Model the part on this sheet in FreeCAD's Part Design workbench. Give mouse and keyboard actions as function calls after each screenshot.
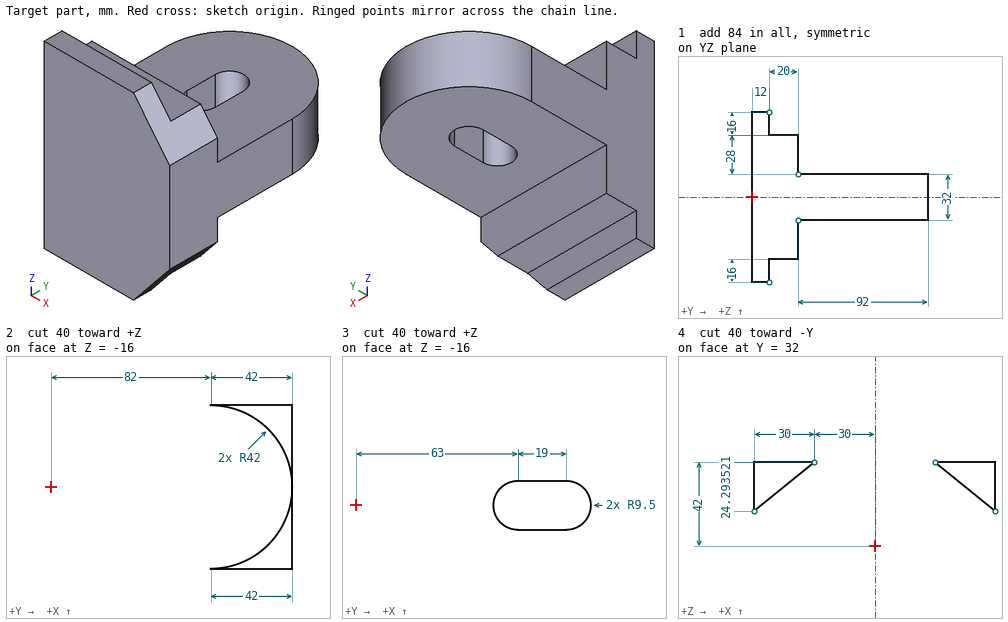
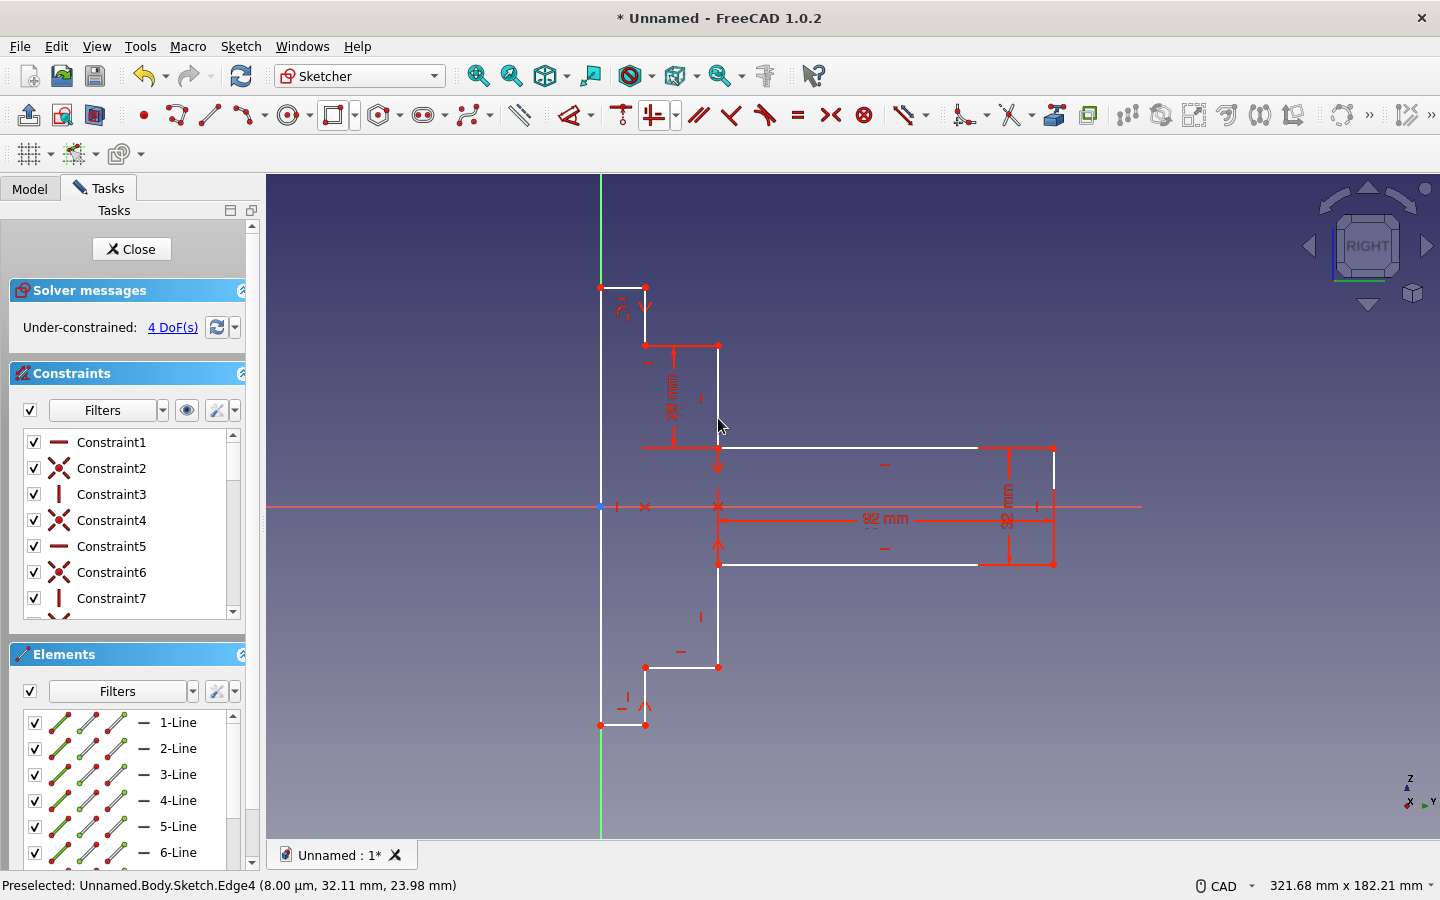
click(696, 346)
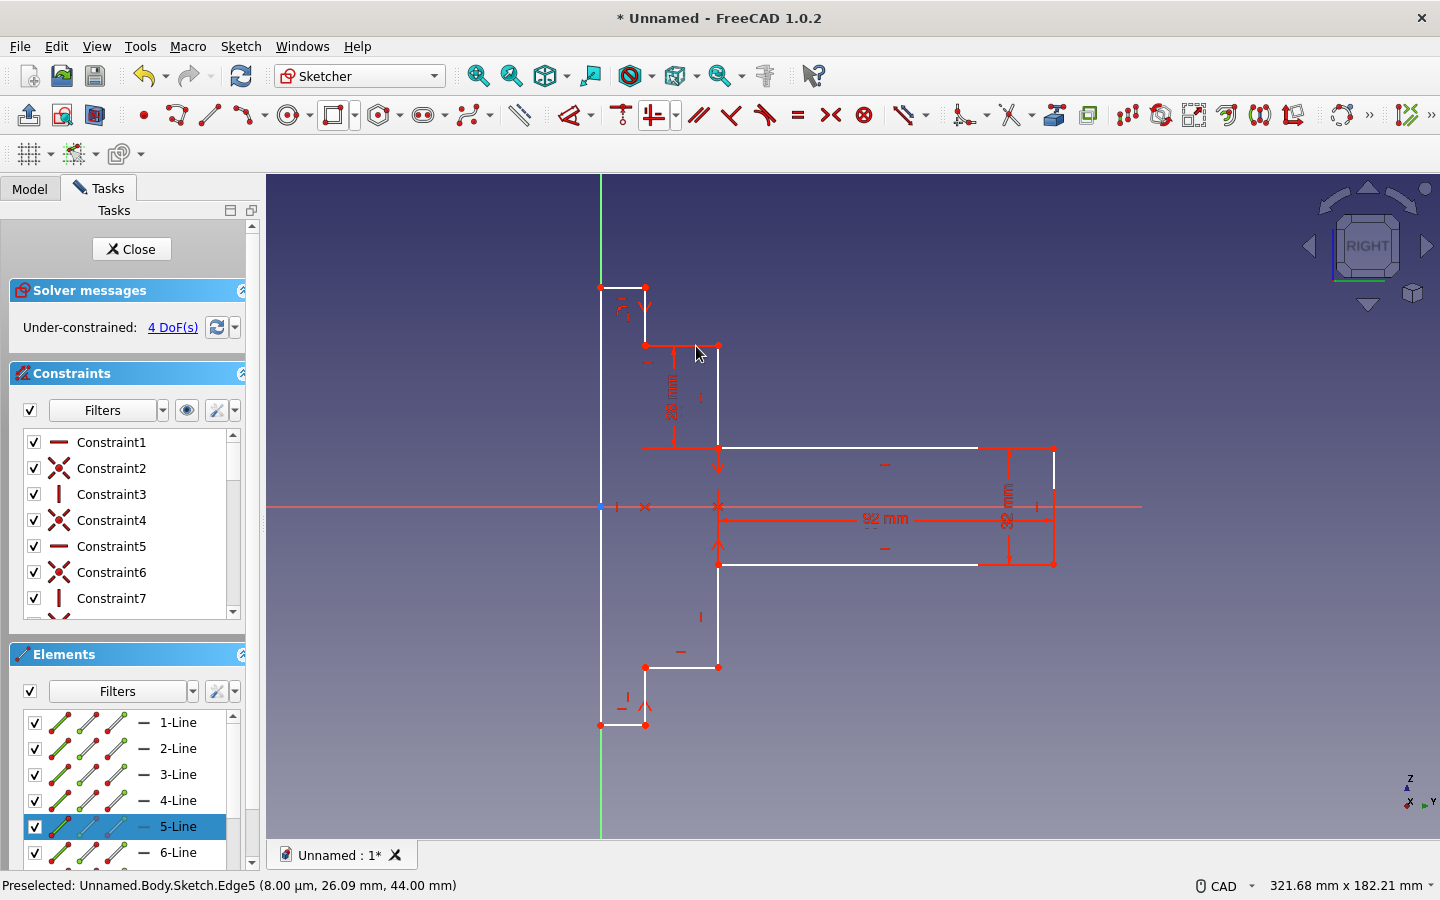
key(l)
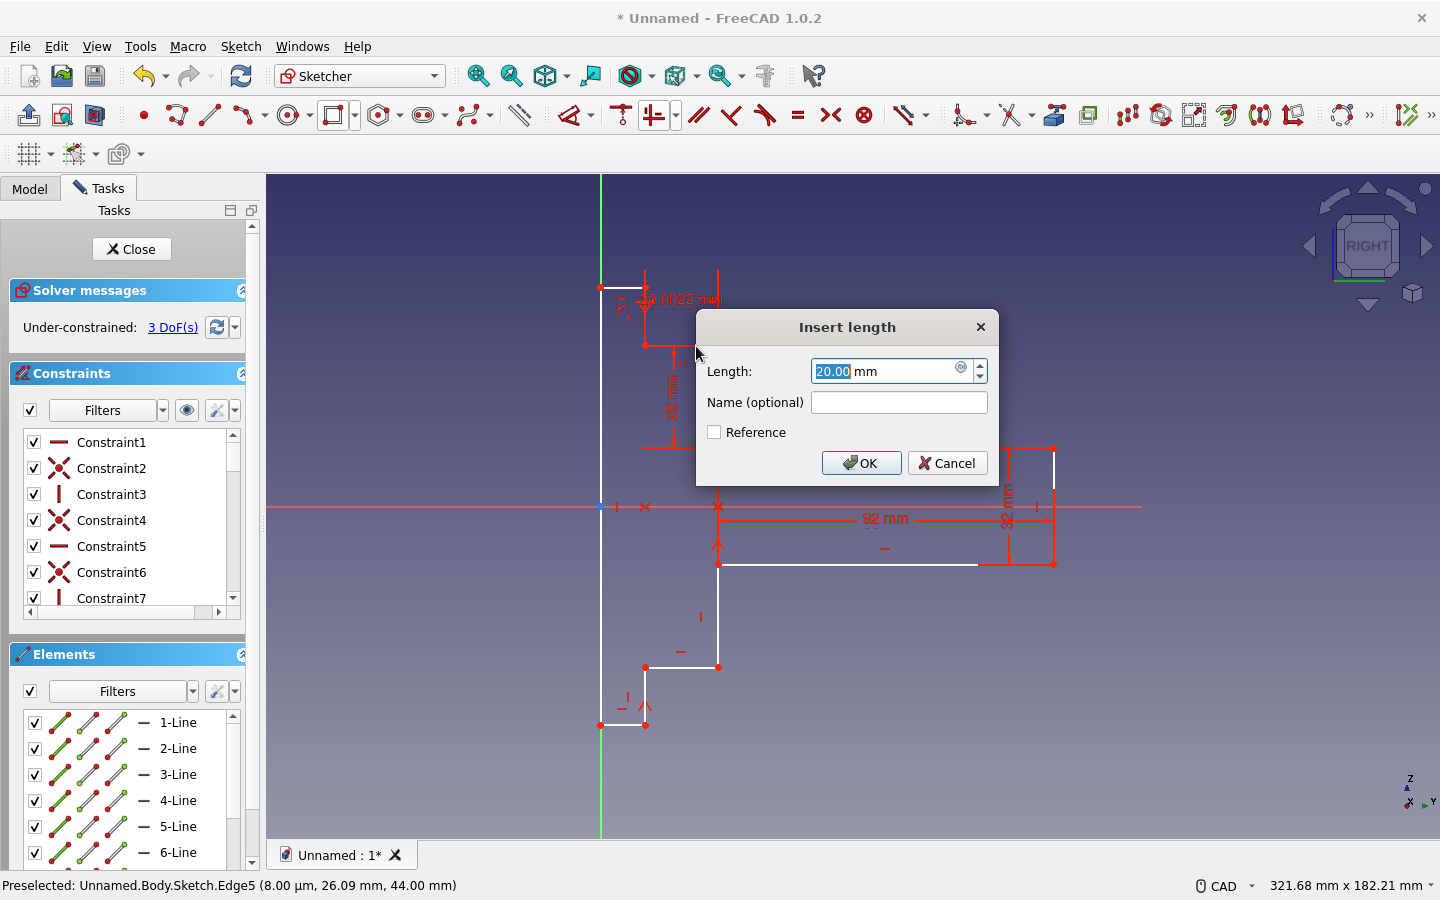
text(20)
key(Return)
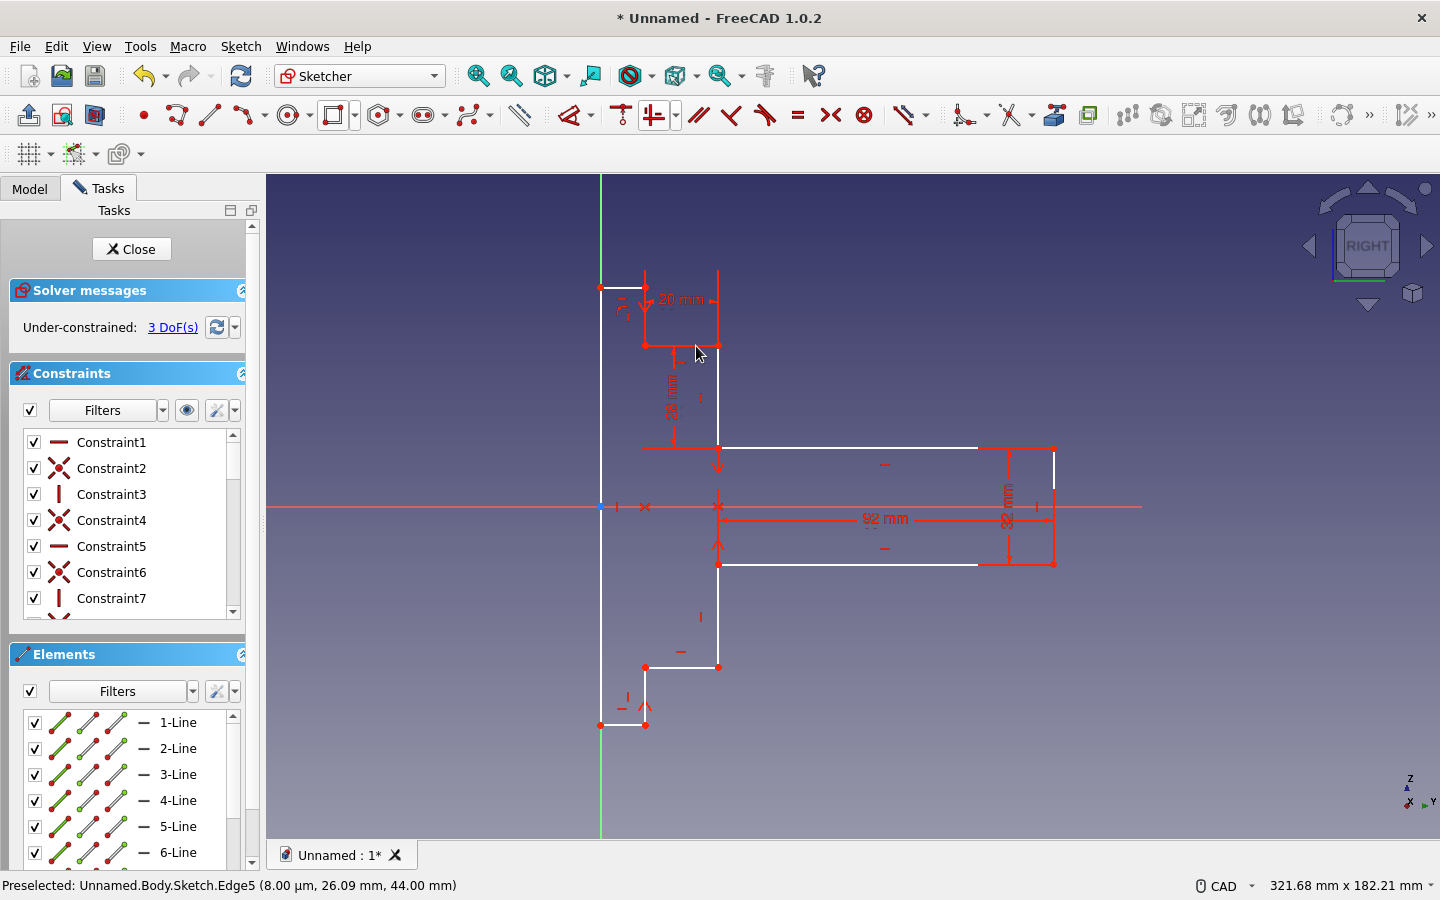
click(645, 328)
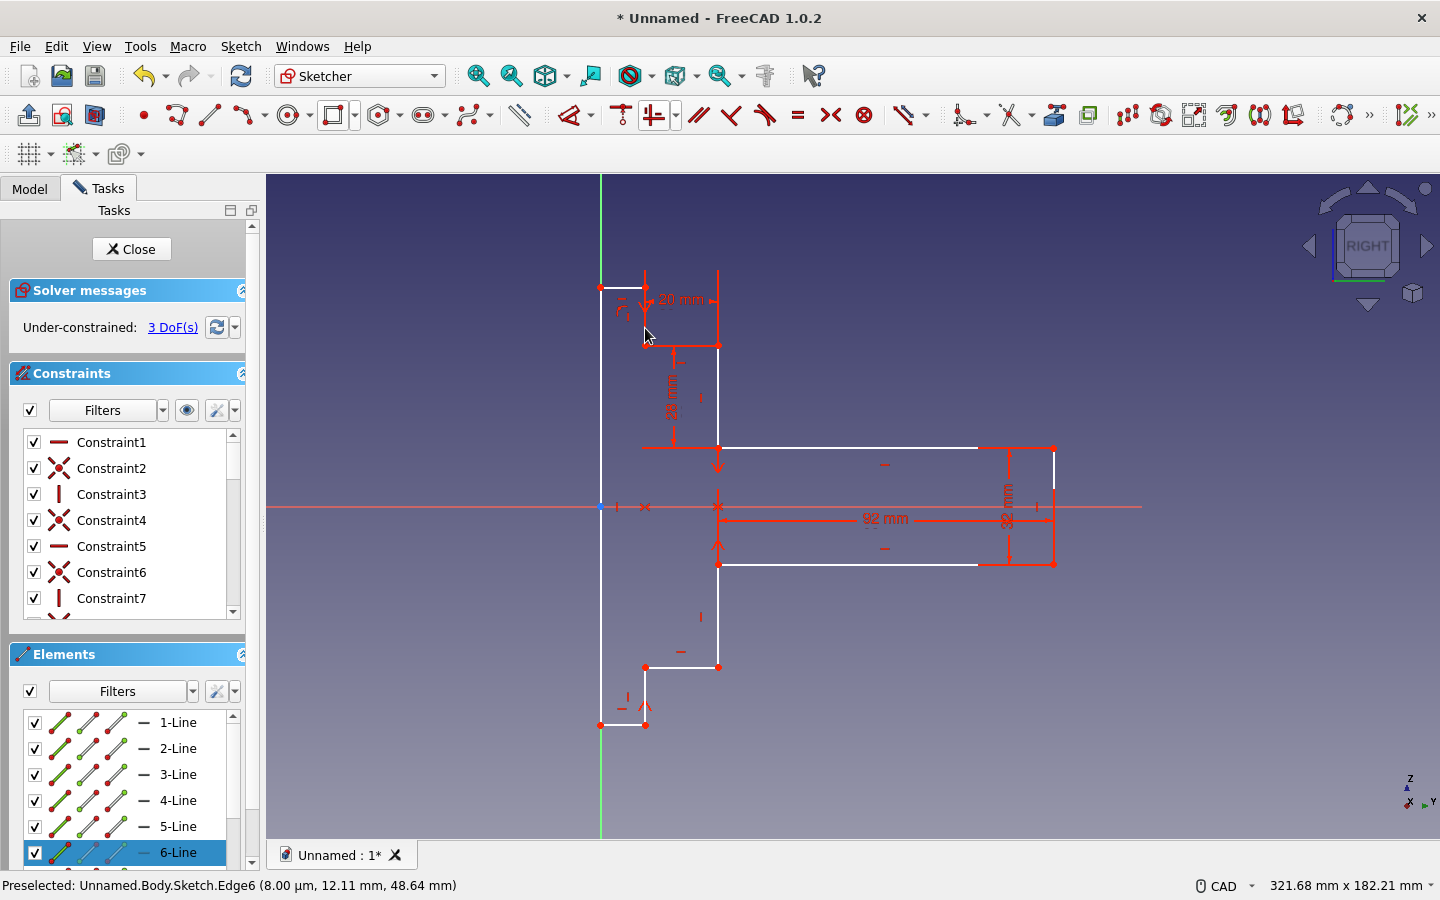
click(590, 116)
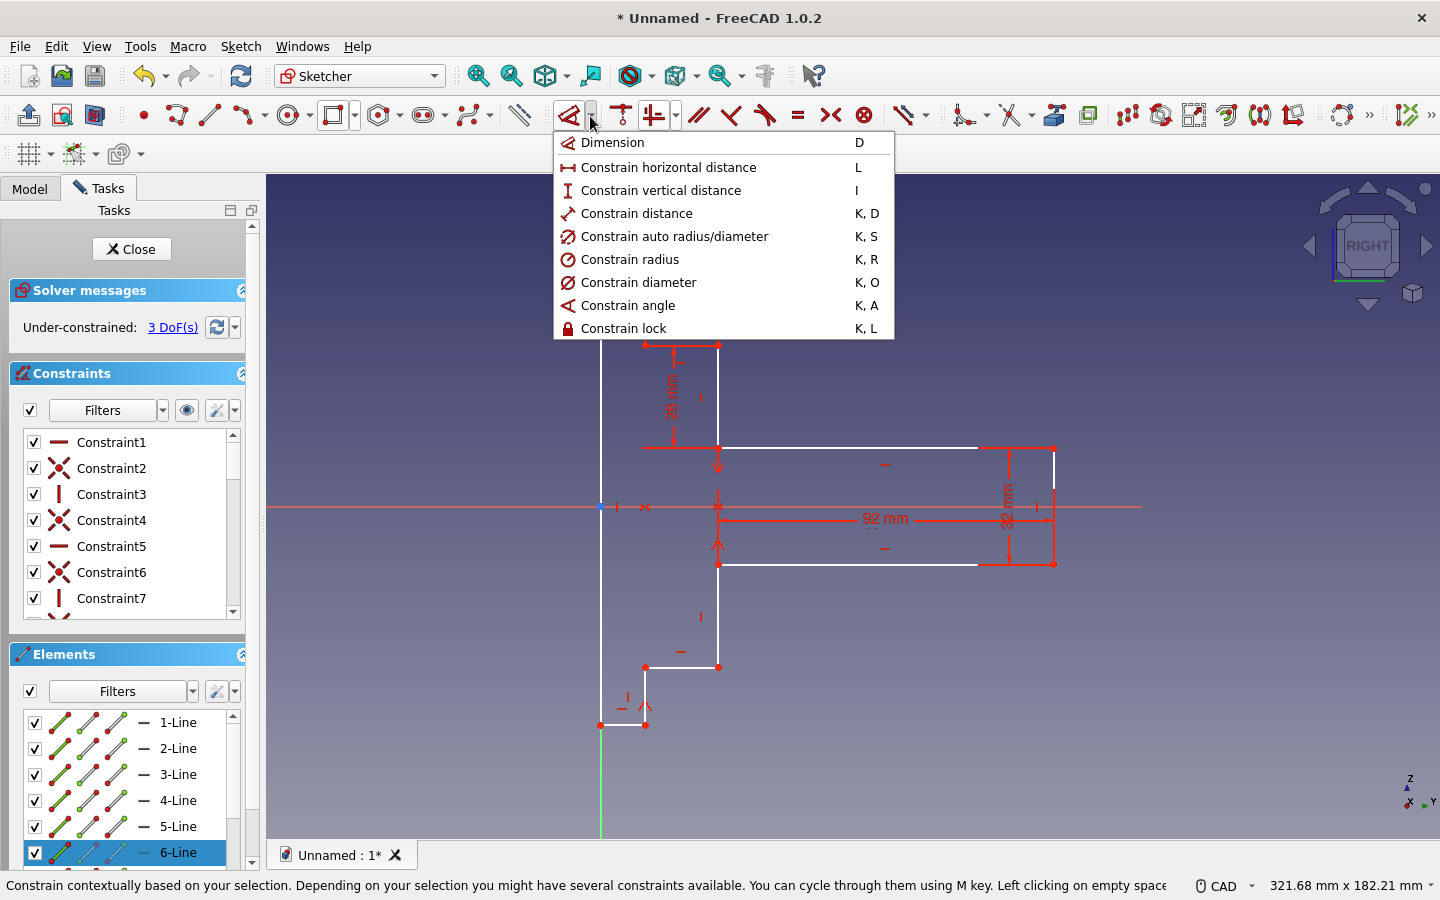
click(724, 190)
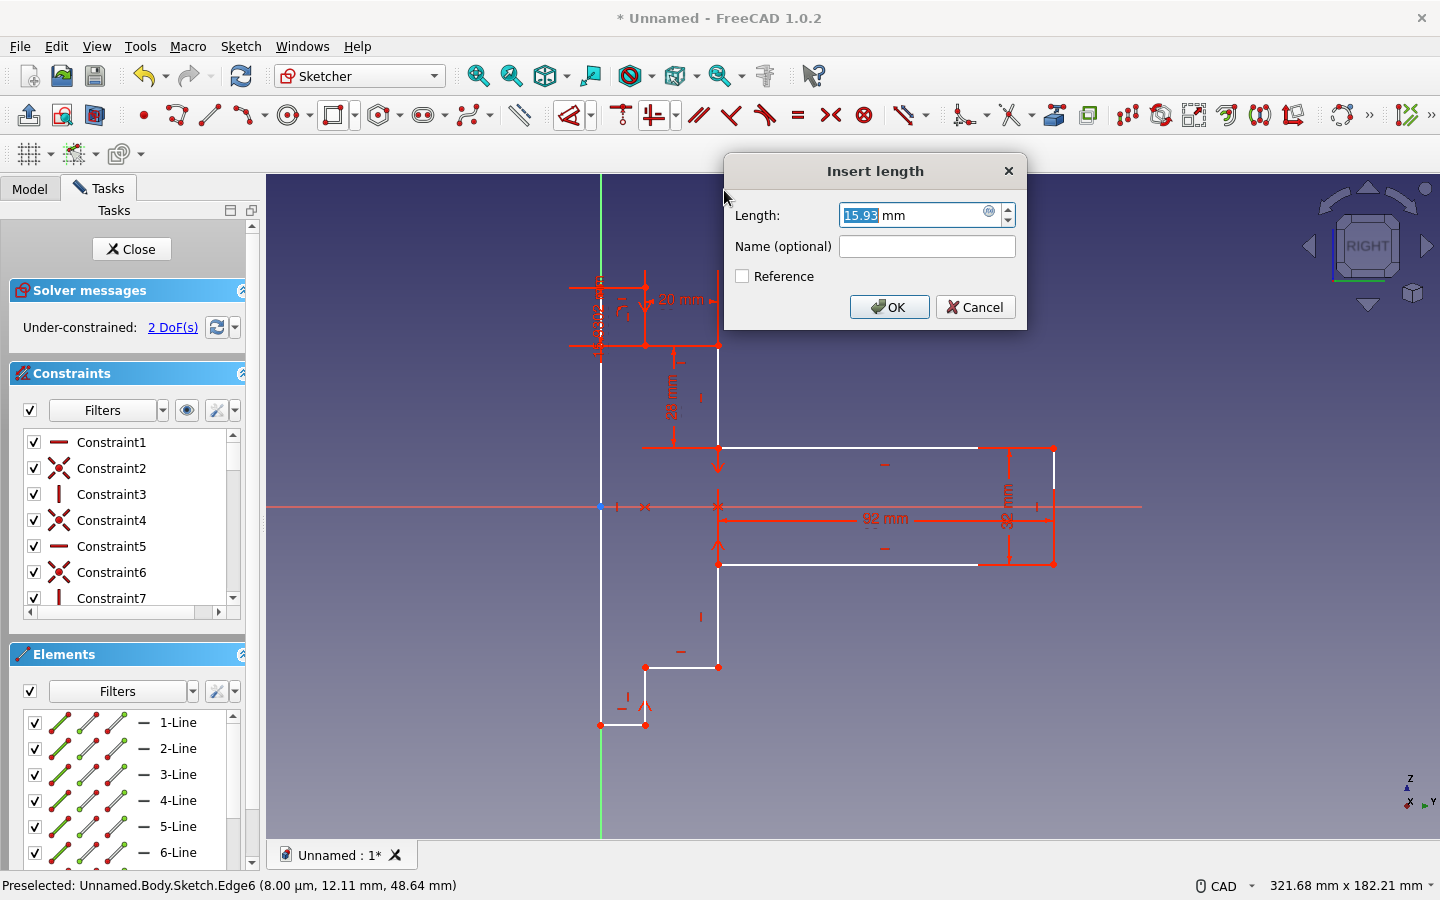
text(16)
key(Return)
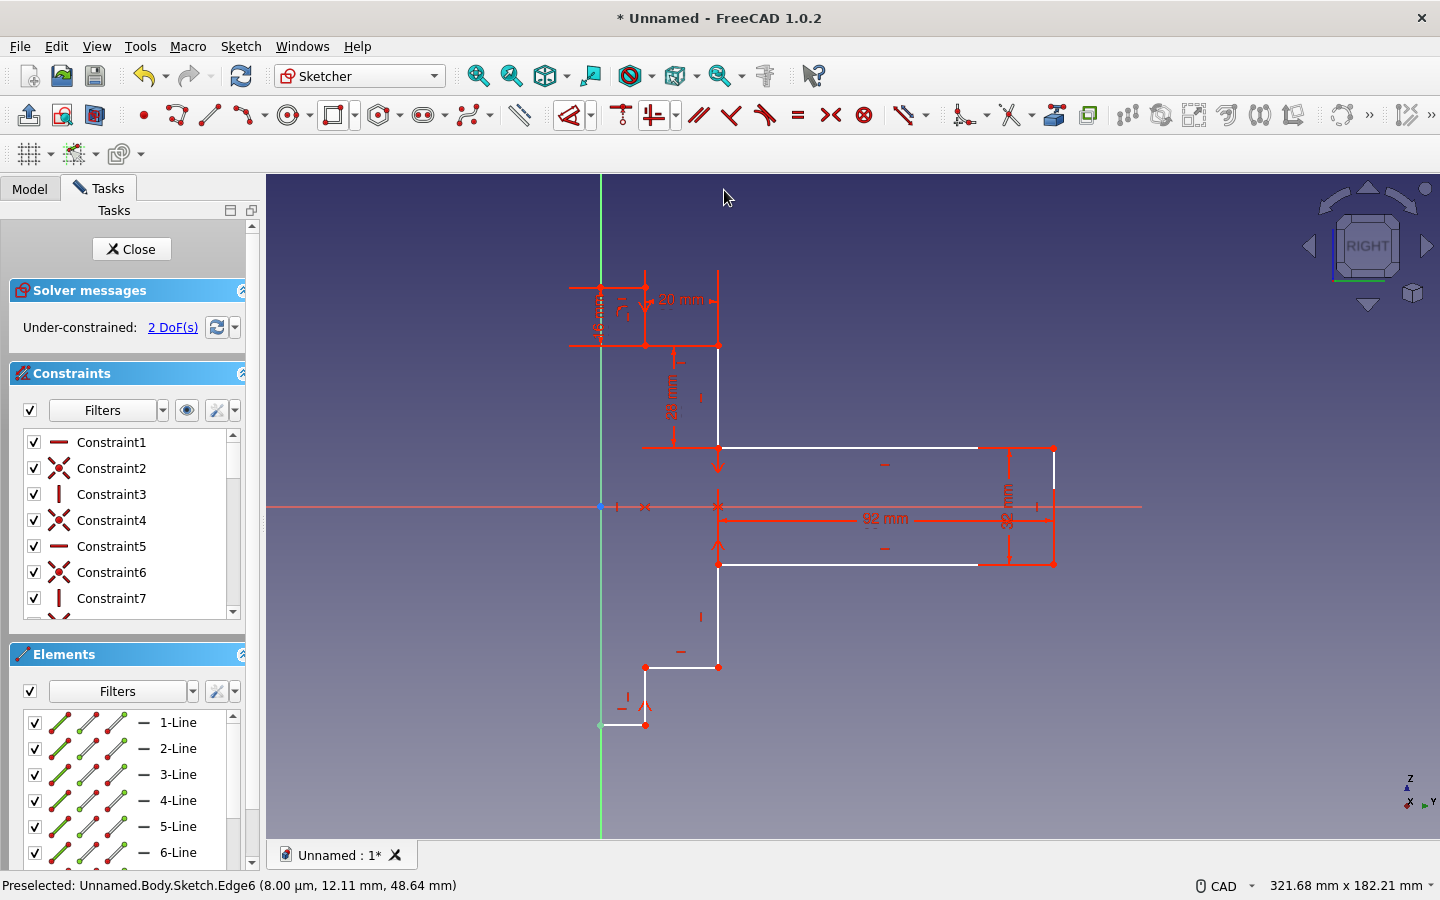
click(632, 288)